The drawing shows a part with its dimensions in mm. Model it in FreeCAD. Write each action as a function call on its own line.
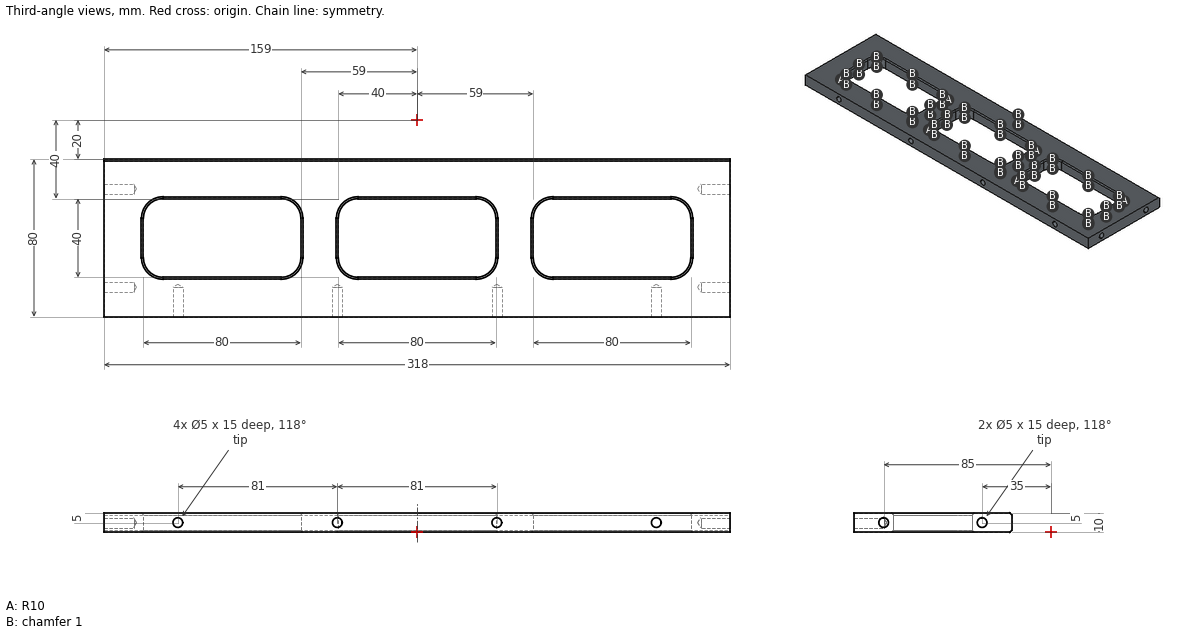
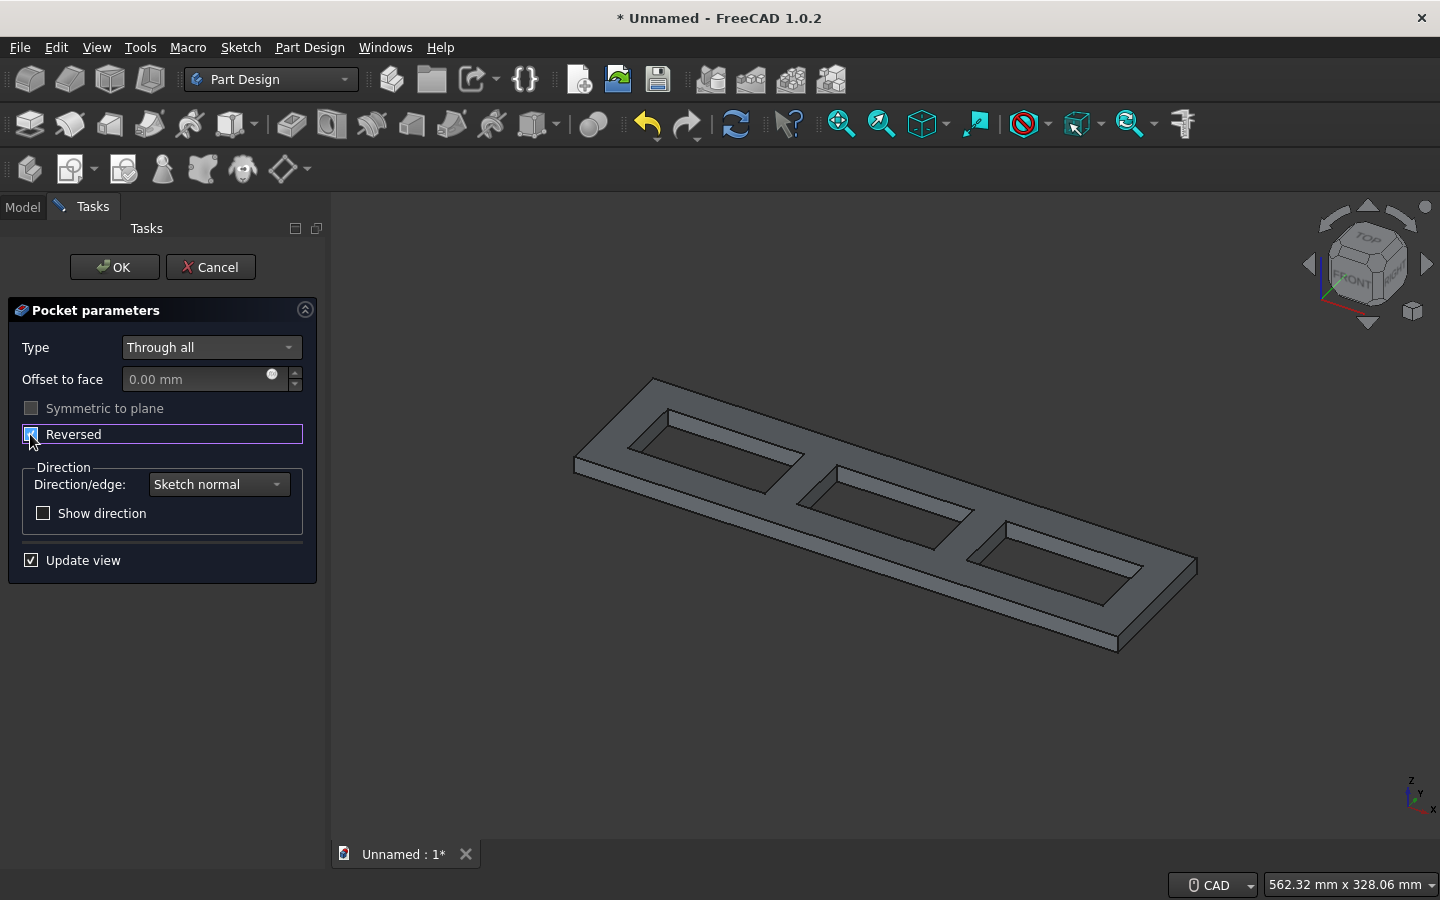
click(115, 267)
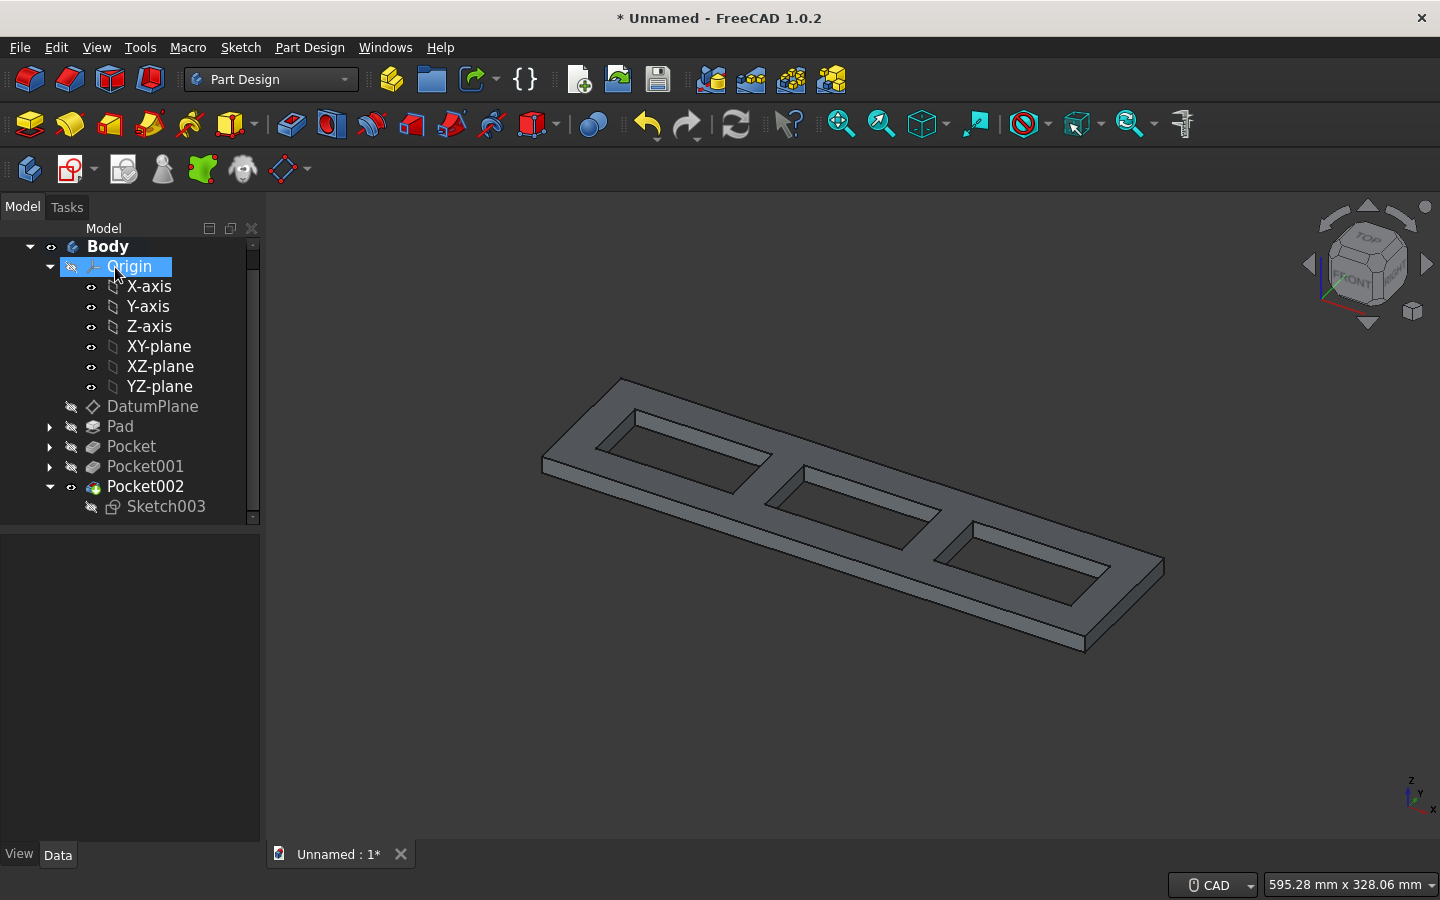
key(6)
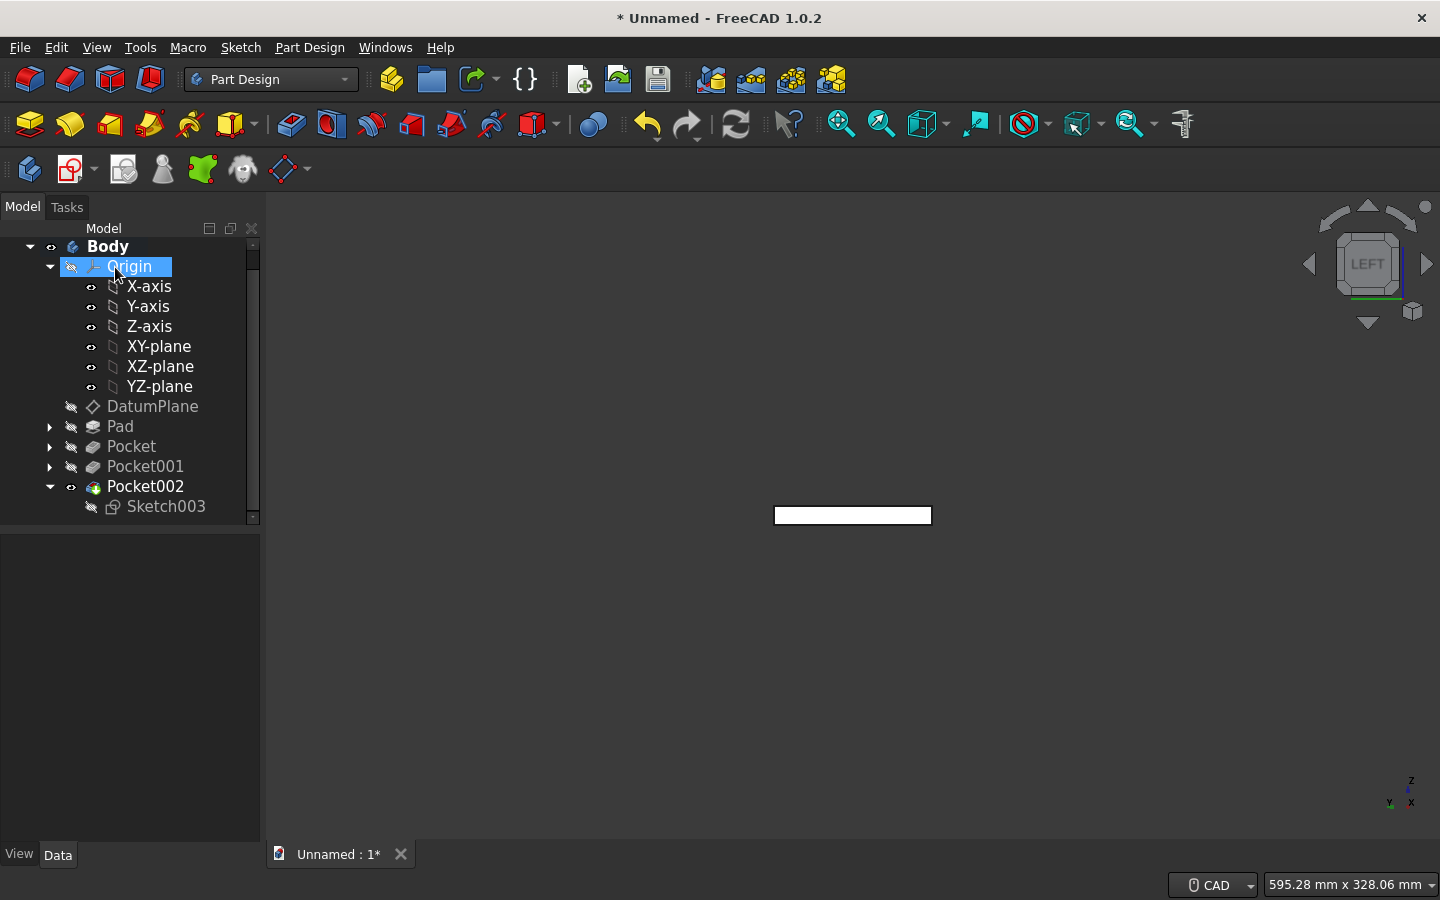
click(842, 124)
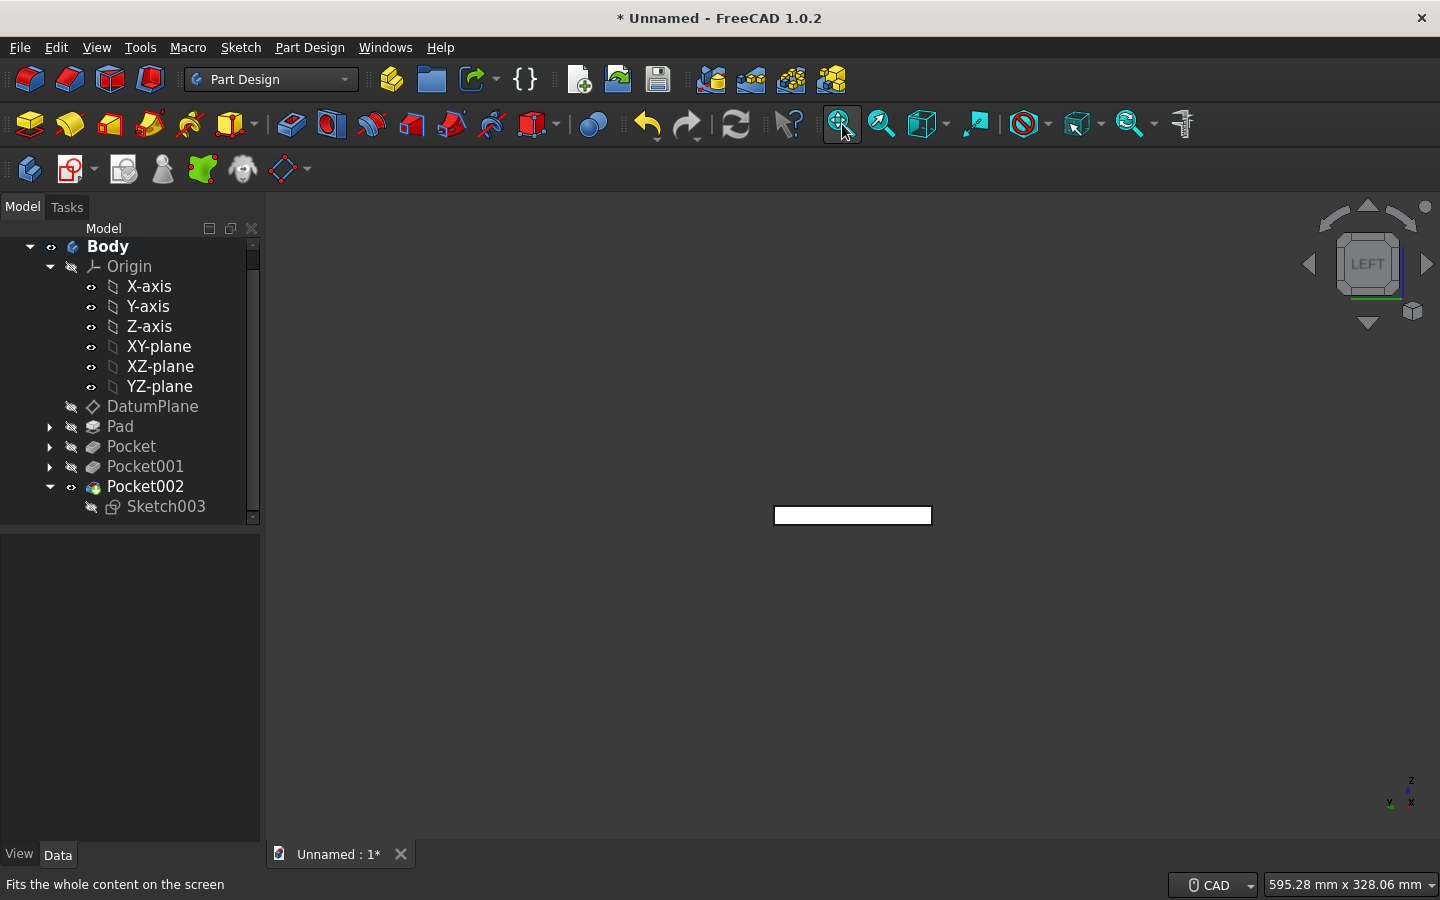
click(785, 514)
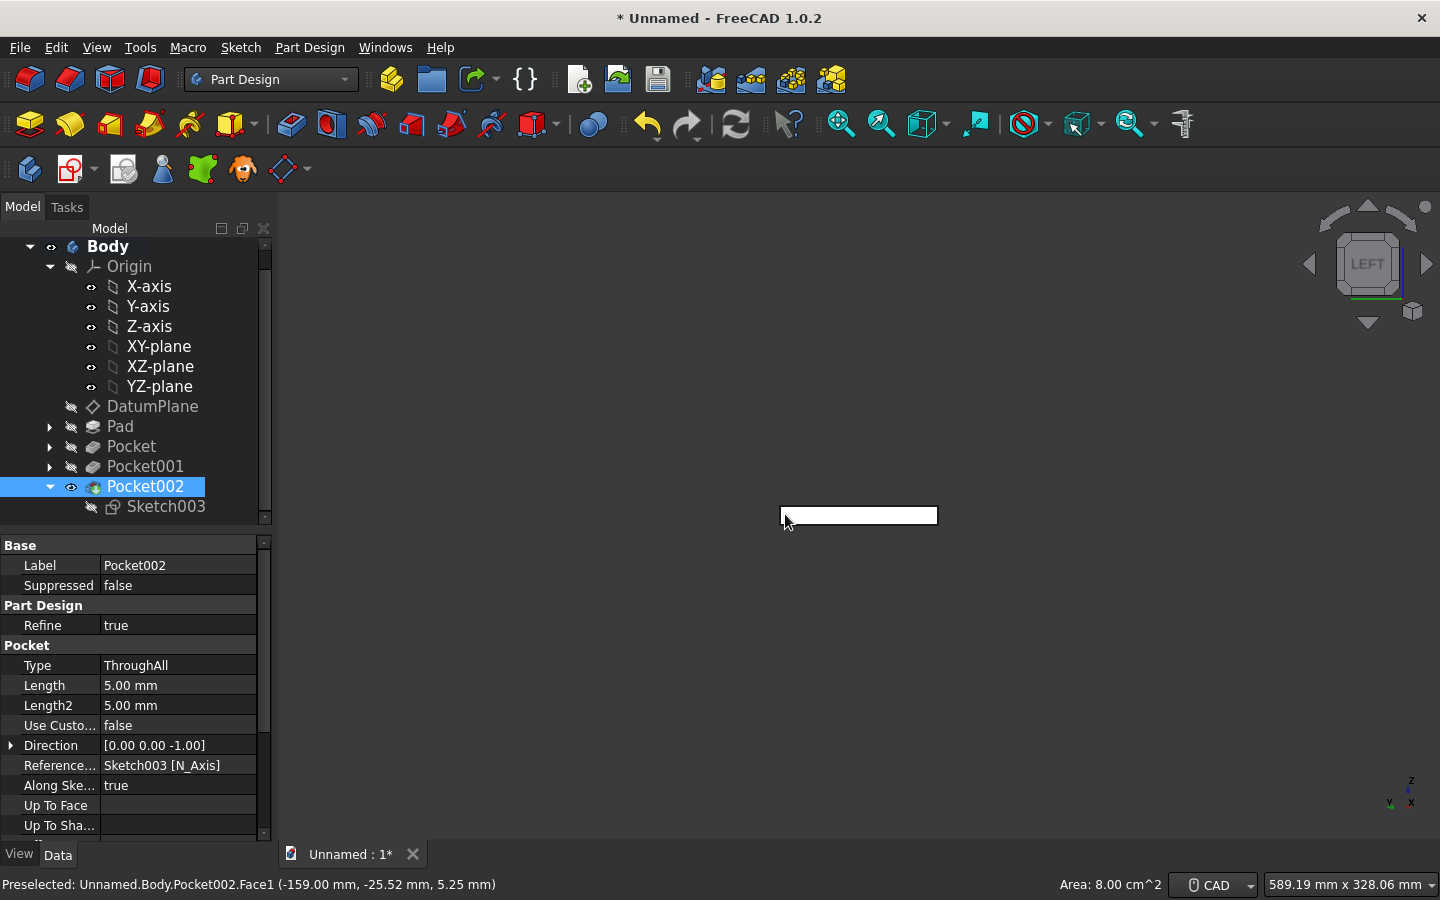
click(70, 170)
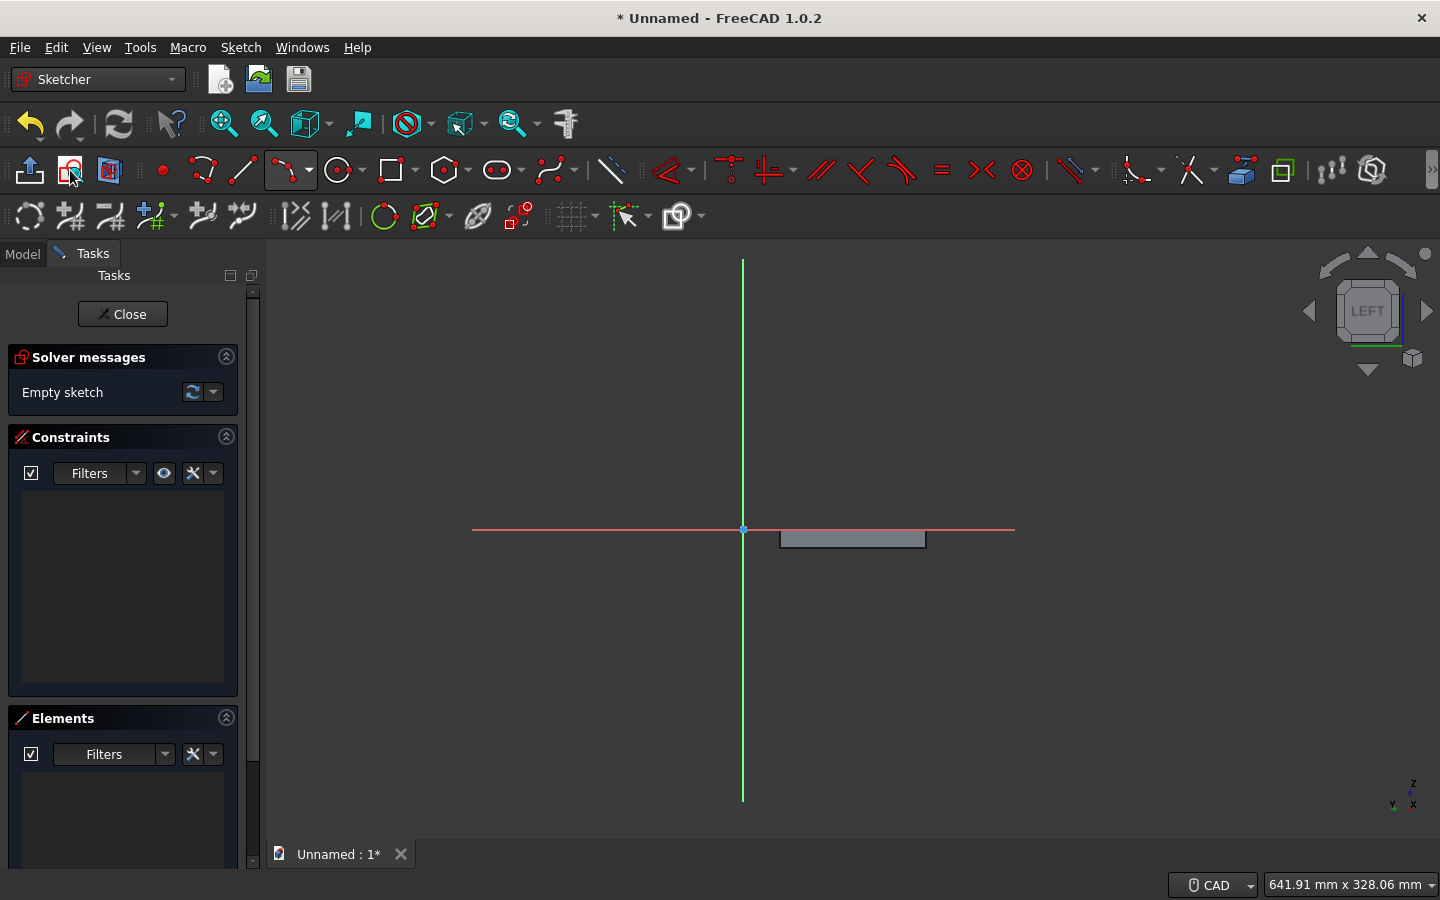
scroll(836, 536, up, 7)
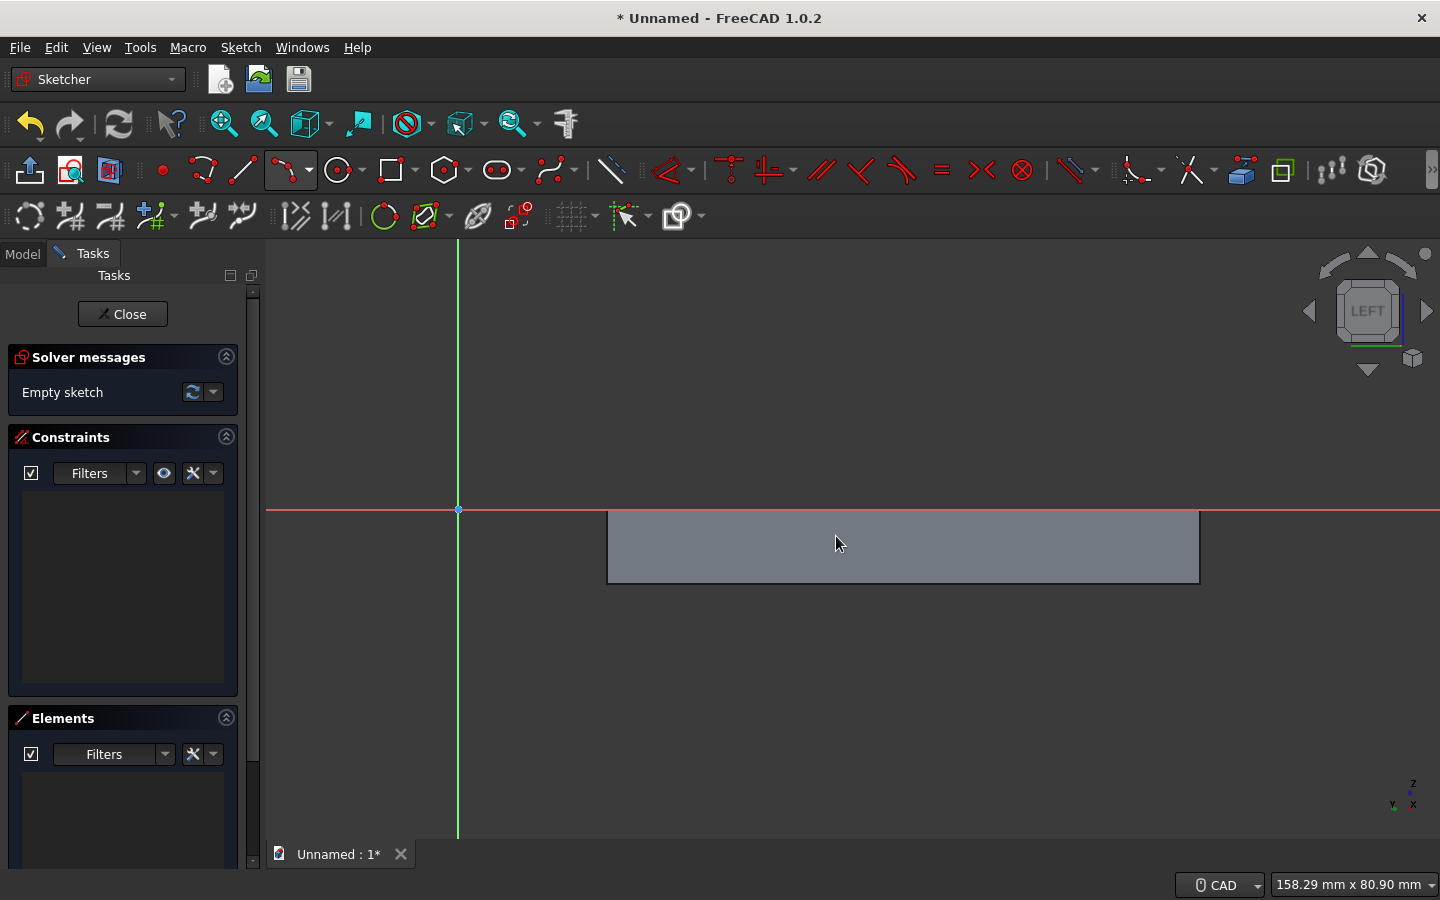
click(338, 170)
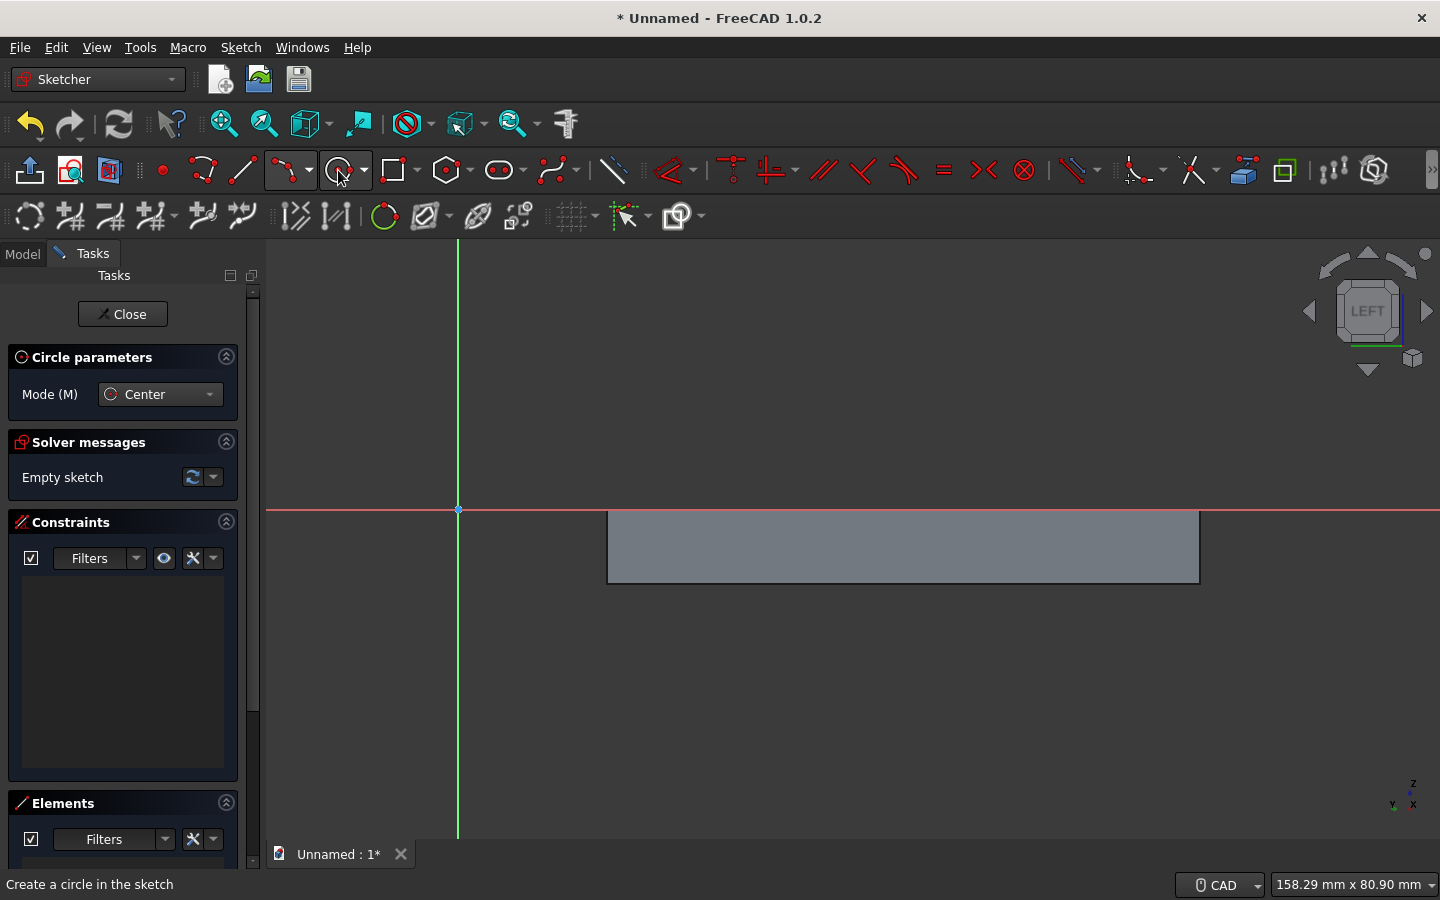
scroll(718, 547, up, 2)